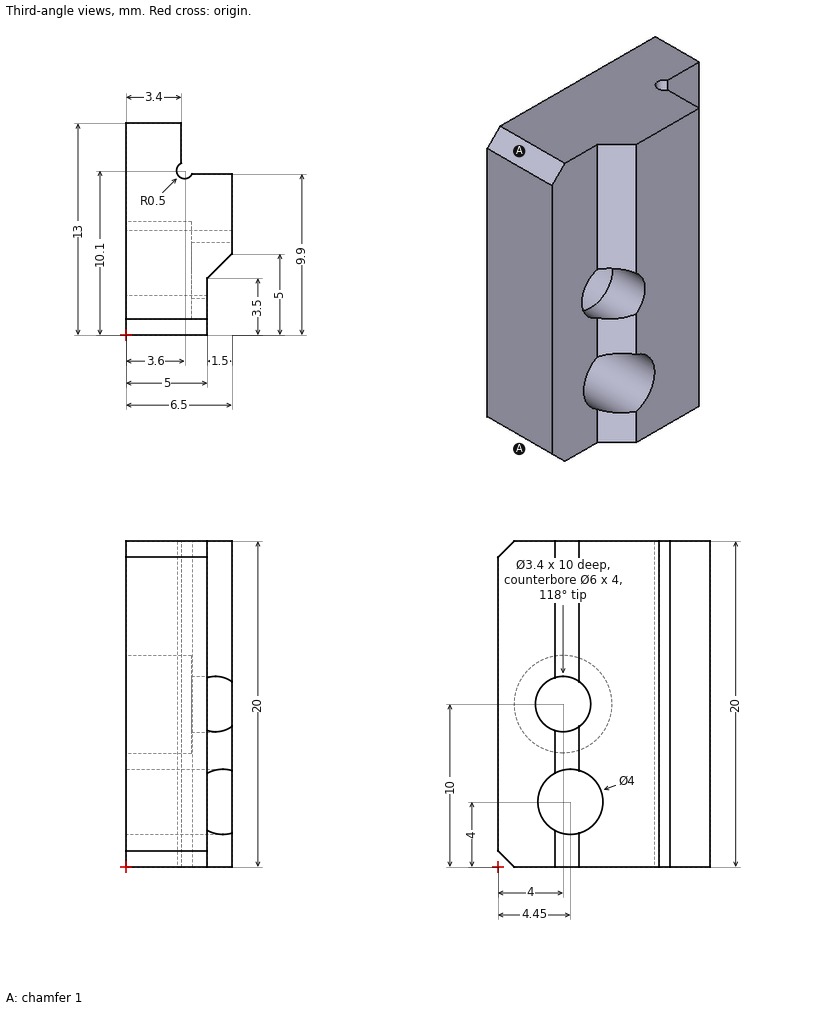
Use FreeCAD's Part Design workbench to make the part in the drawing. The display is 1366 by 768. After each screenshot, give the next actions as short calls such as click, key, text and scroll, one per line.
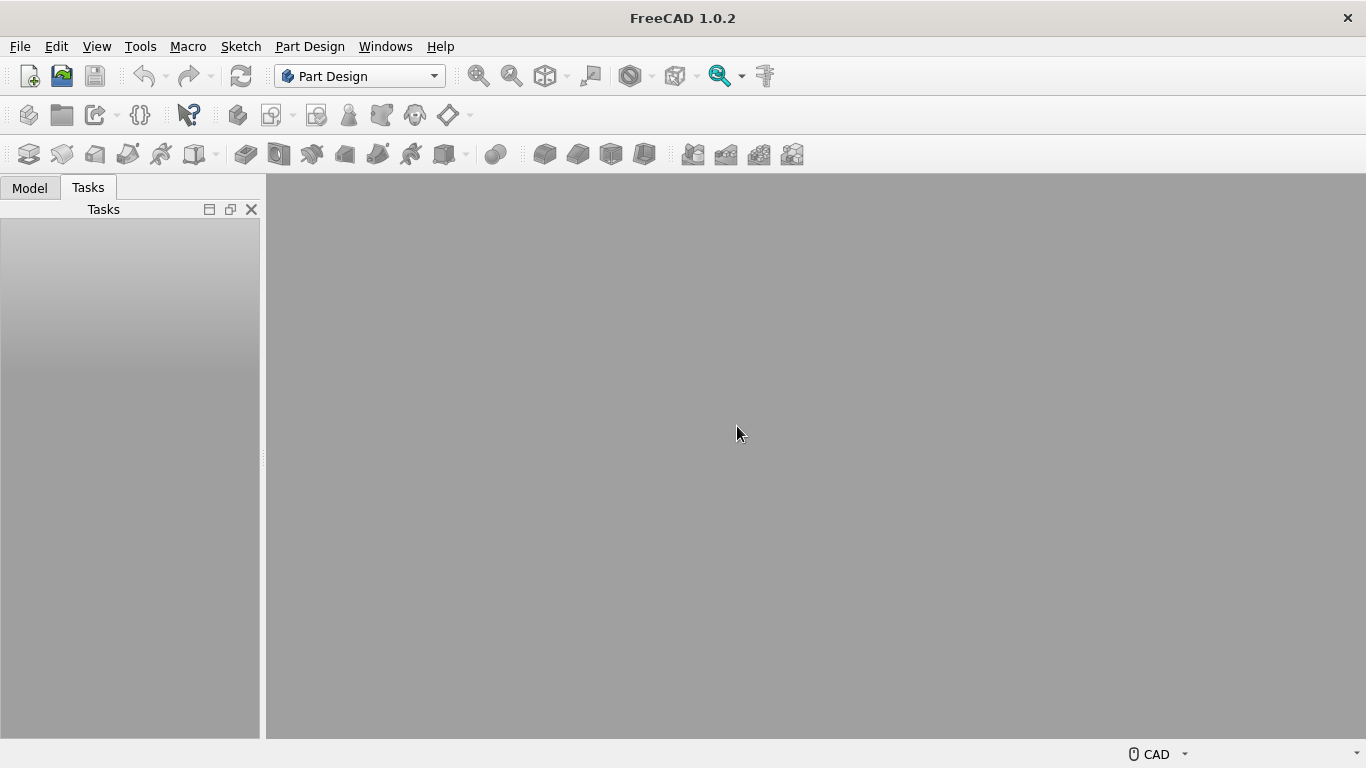
click(29, 76)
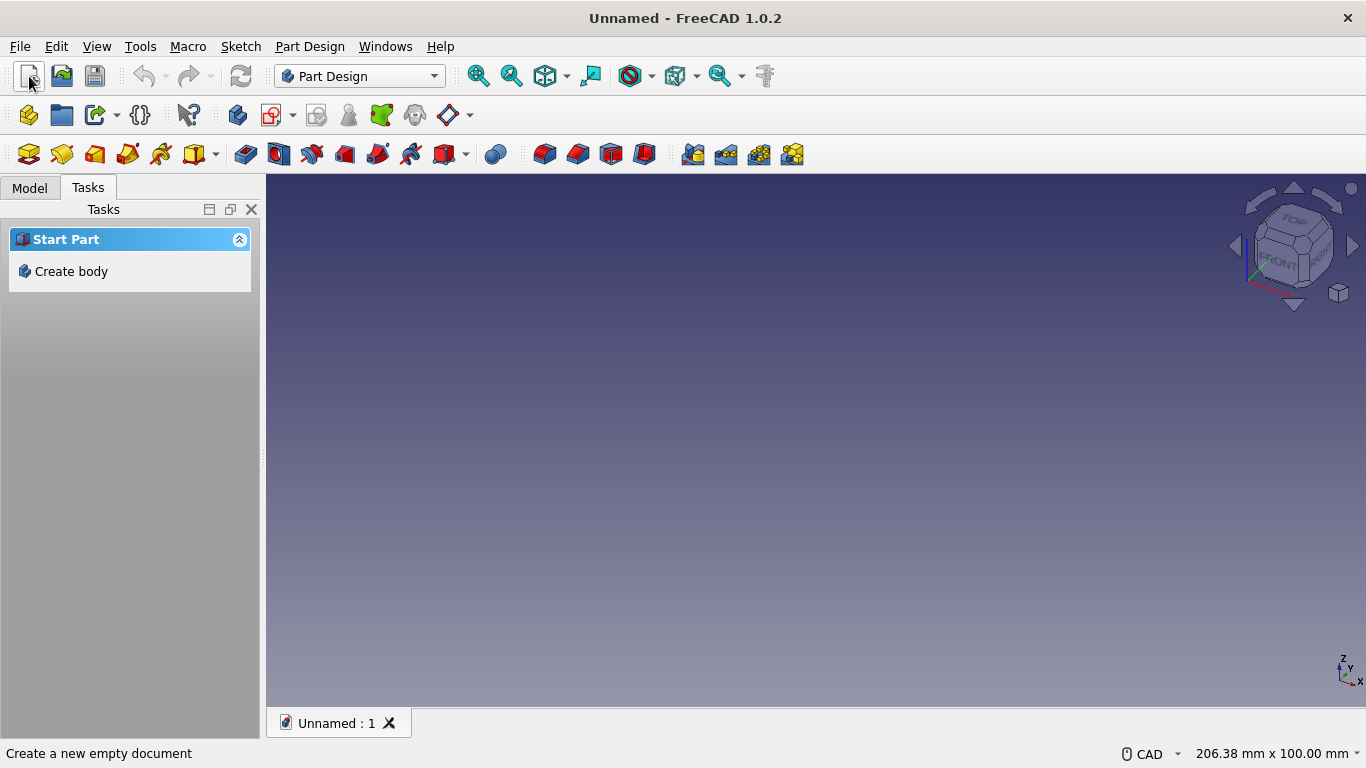
click(270, 116)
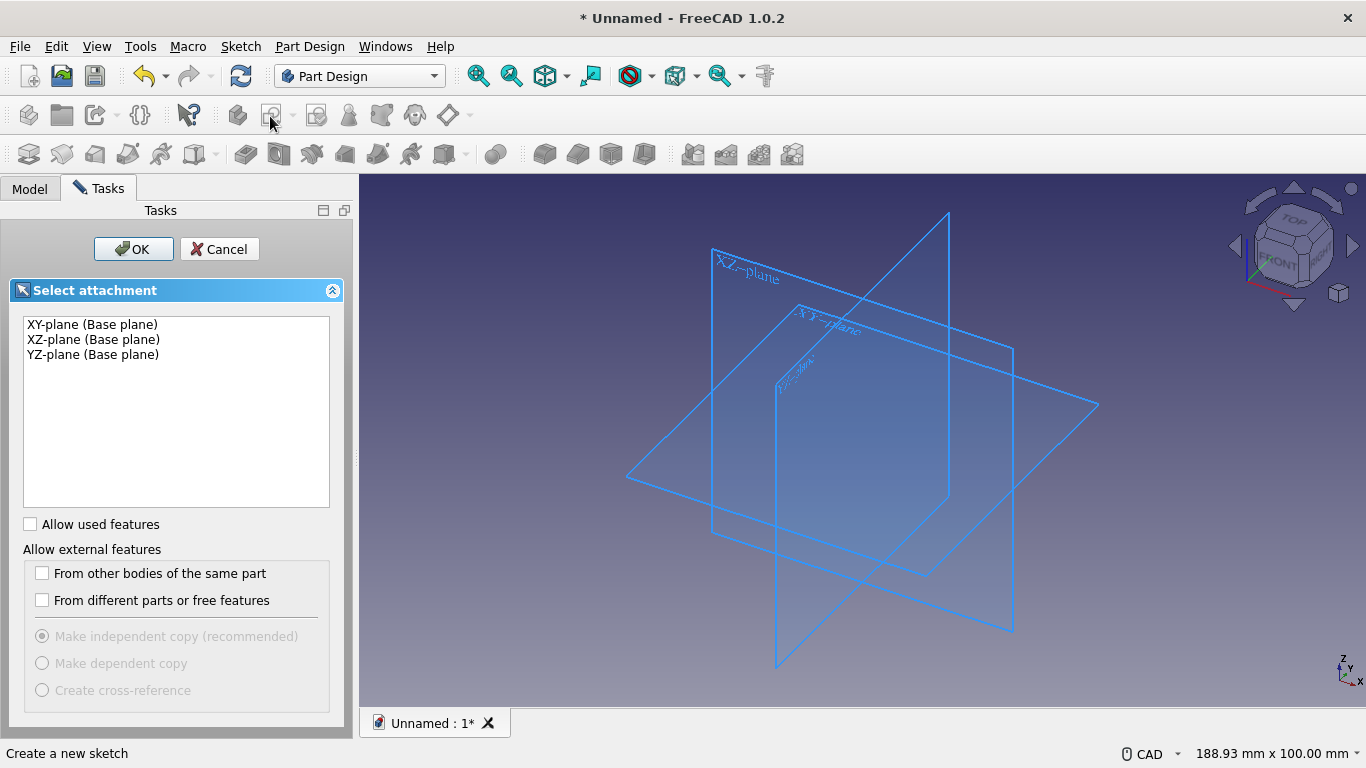
click(84, 324)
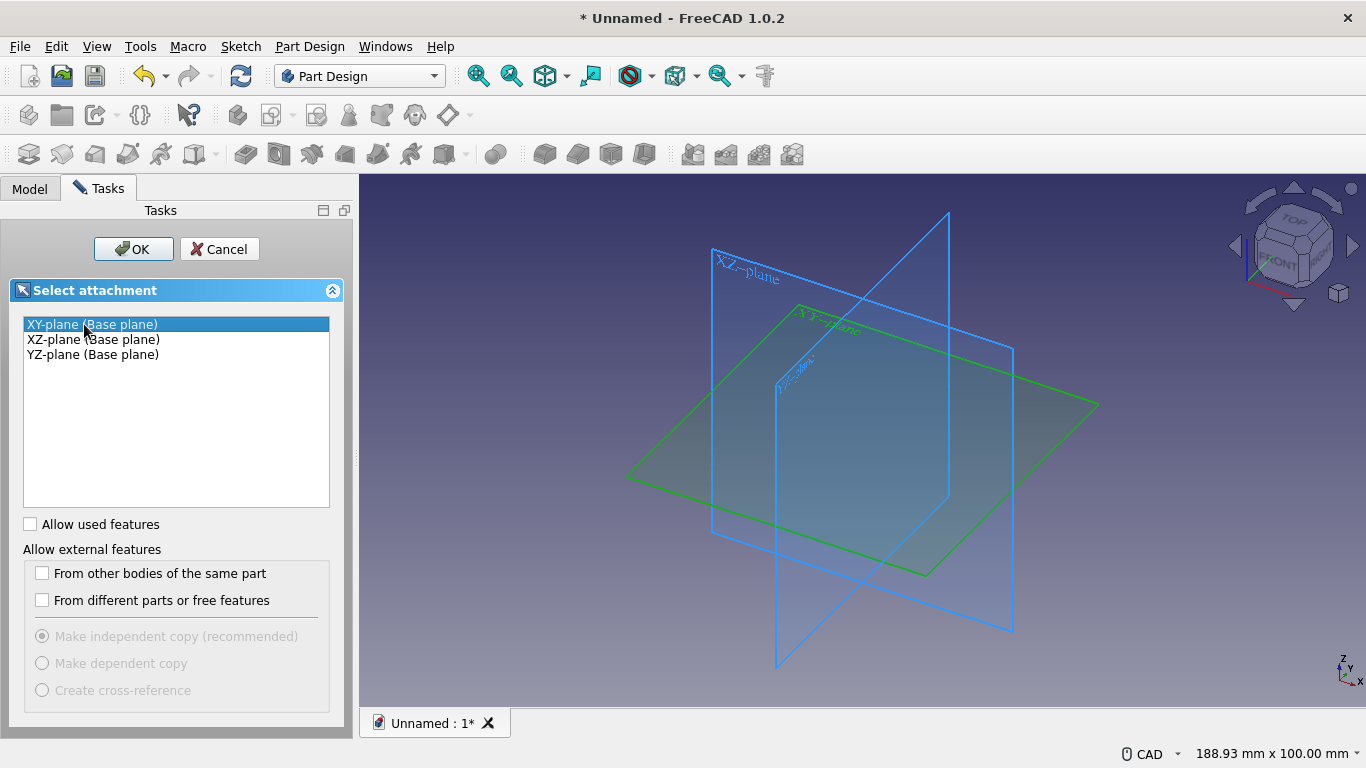
click(134, 249)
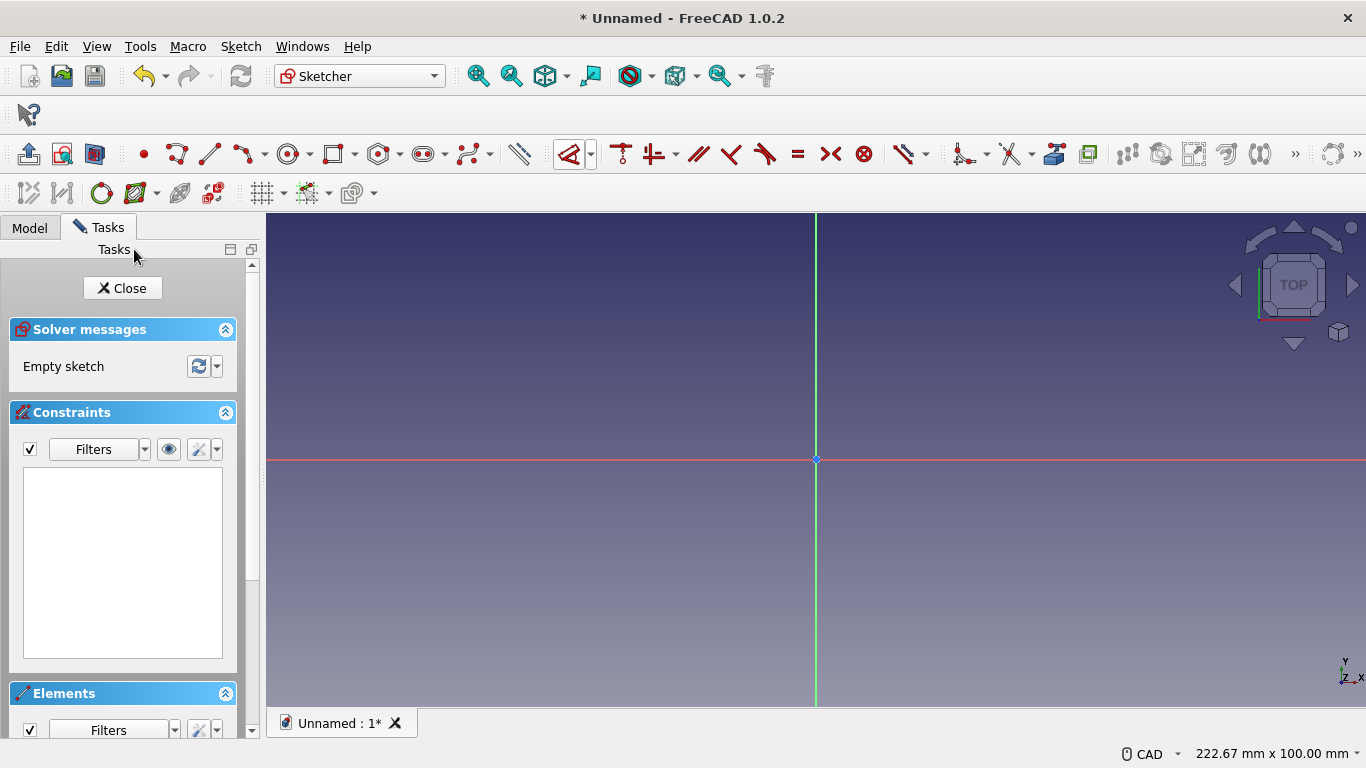
scroll(853, 420, up, 8)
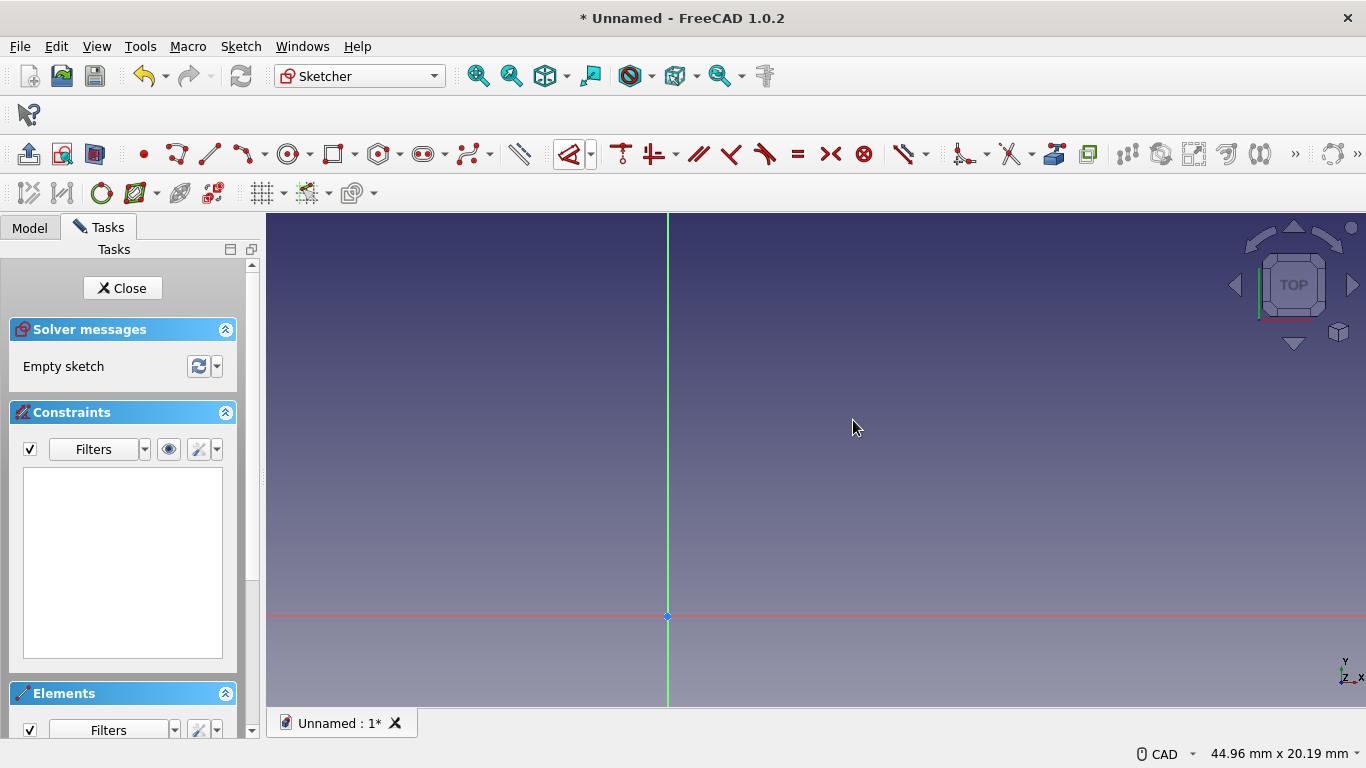
click(177, 154)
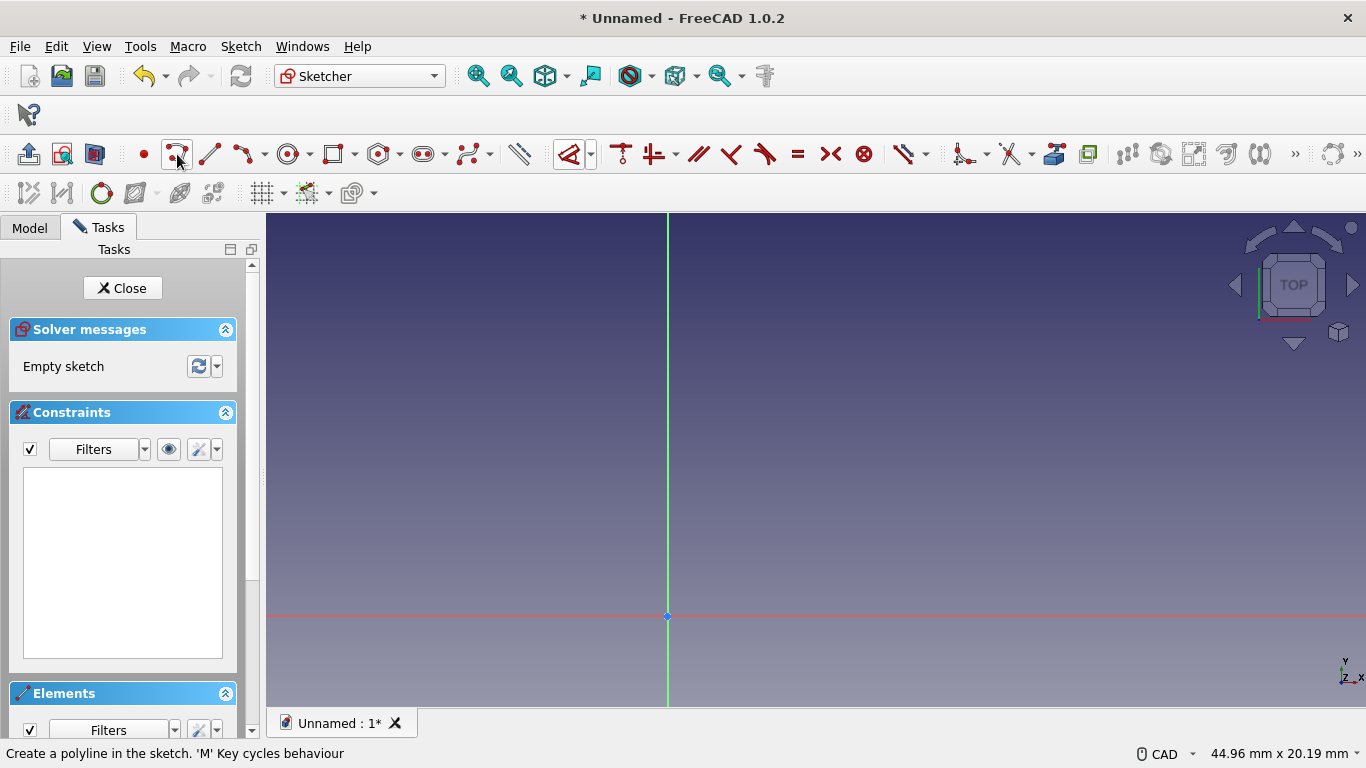
click(751, 358)
click(751, 298)
click(668, 298)
click(668, 616)
click(827, 607)
click(827, 374)
click(767, 374)
right_click(767, 374)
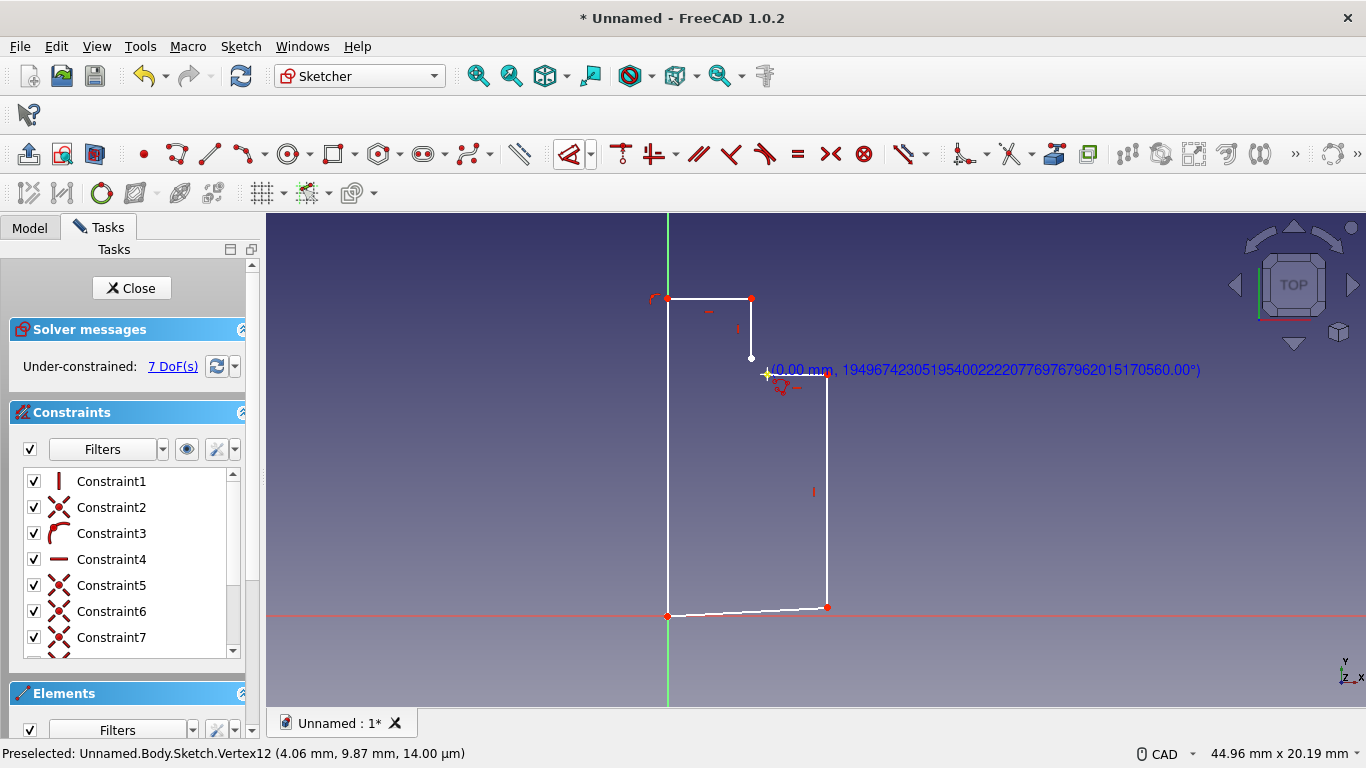
click(242, 154)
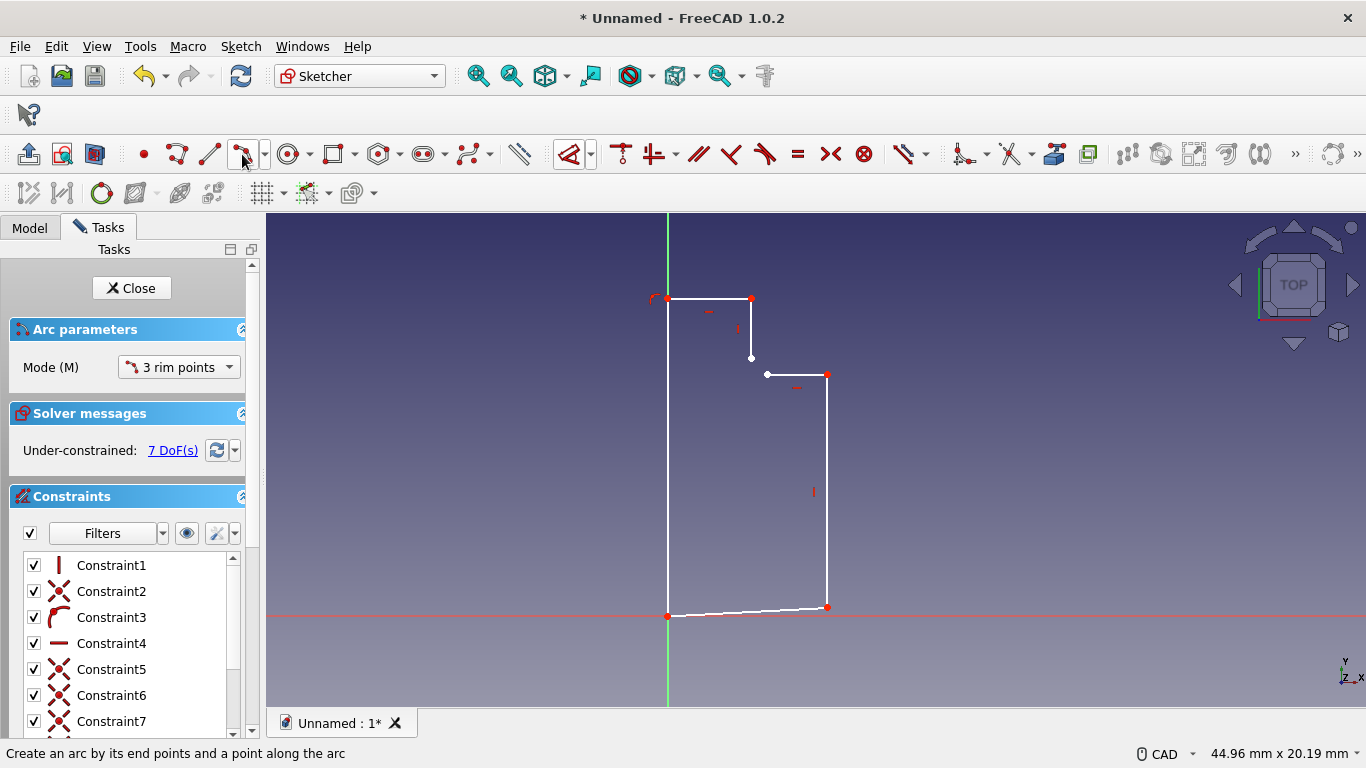
click(767, 375)
click(751, 359)
click(747, 378)
key(Escape)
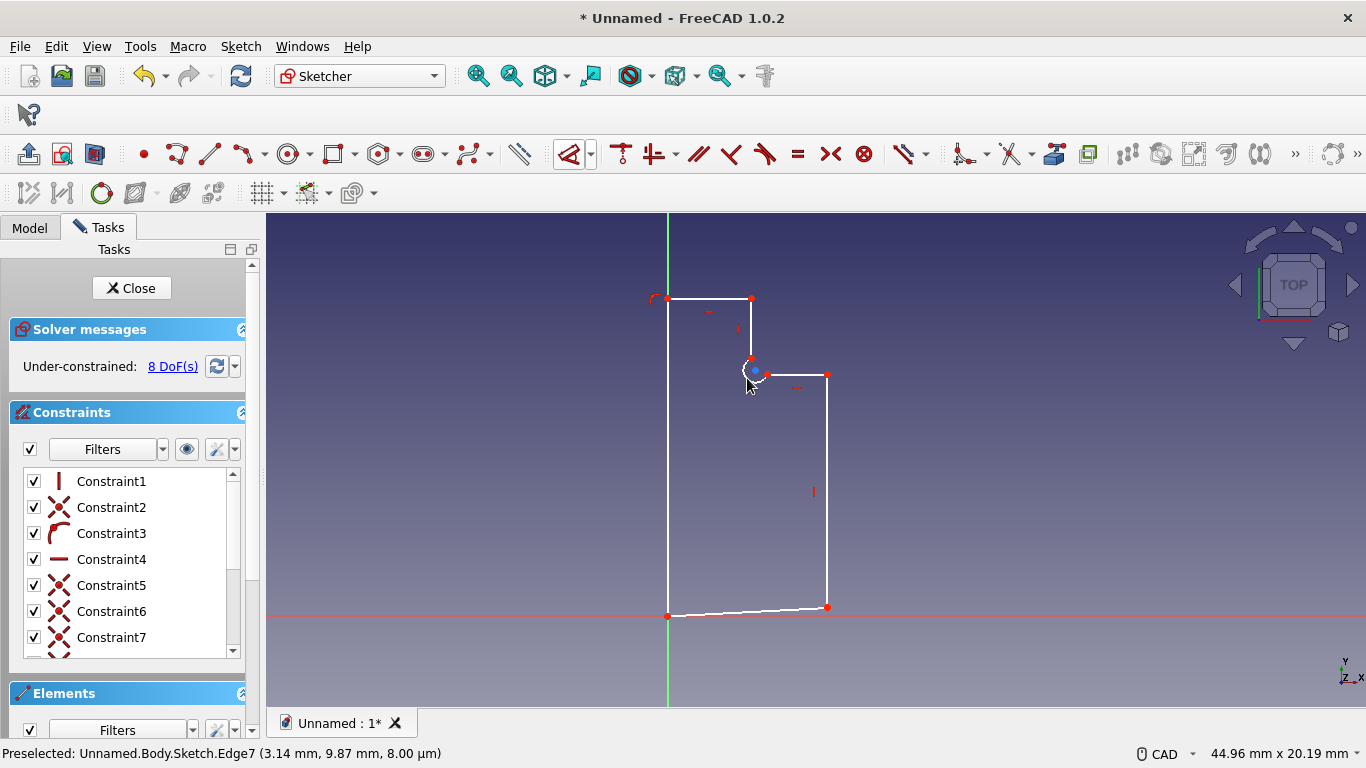
click(715, 614)